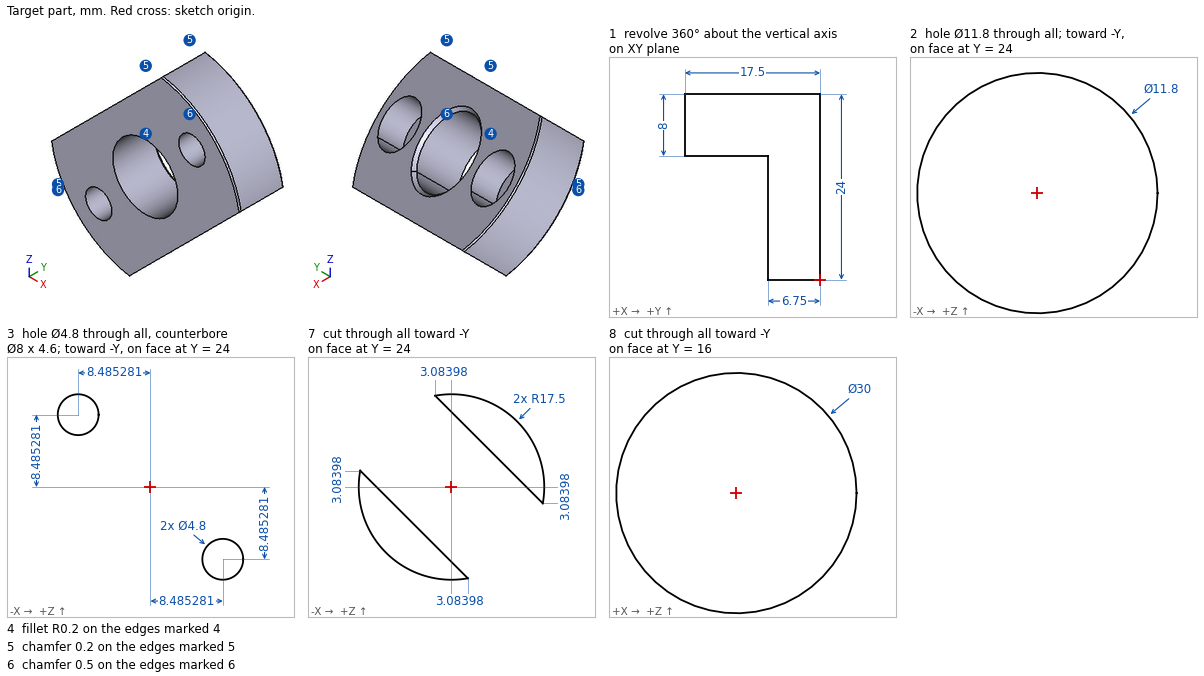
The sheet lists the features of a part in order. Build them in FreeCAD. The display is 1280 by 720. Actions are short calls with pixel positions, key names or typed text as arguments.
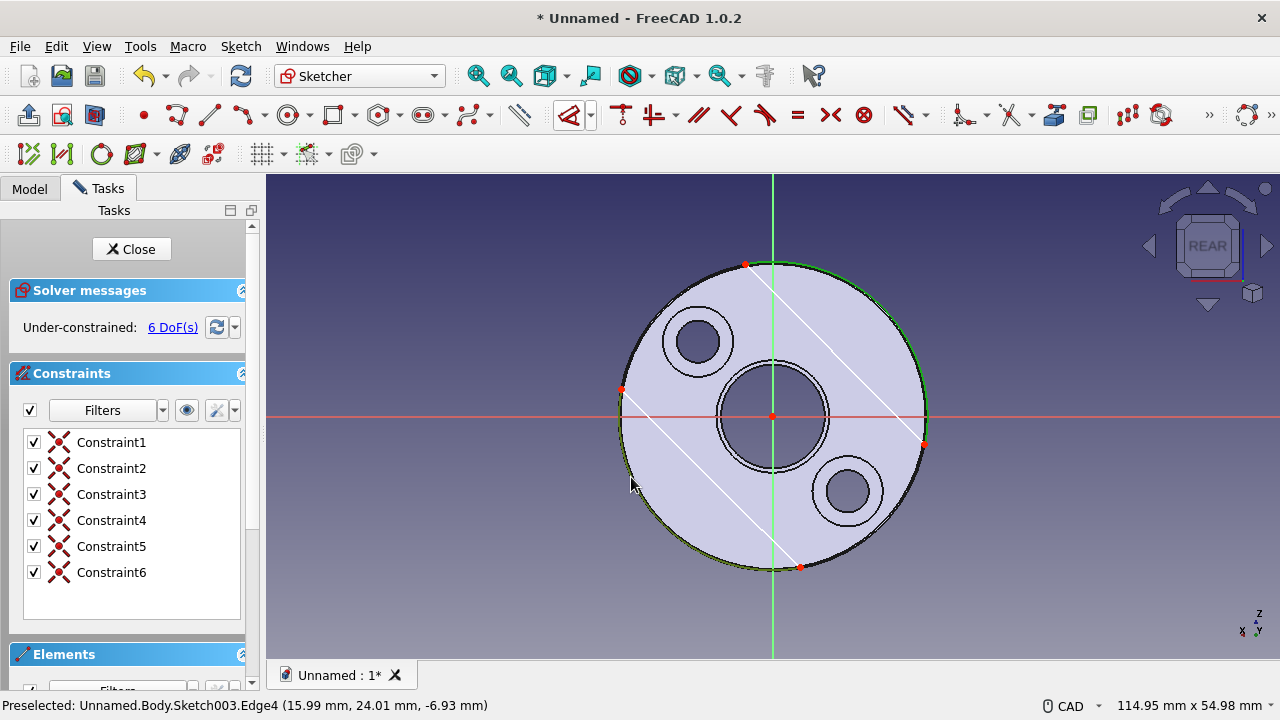
click(798, 116)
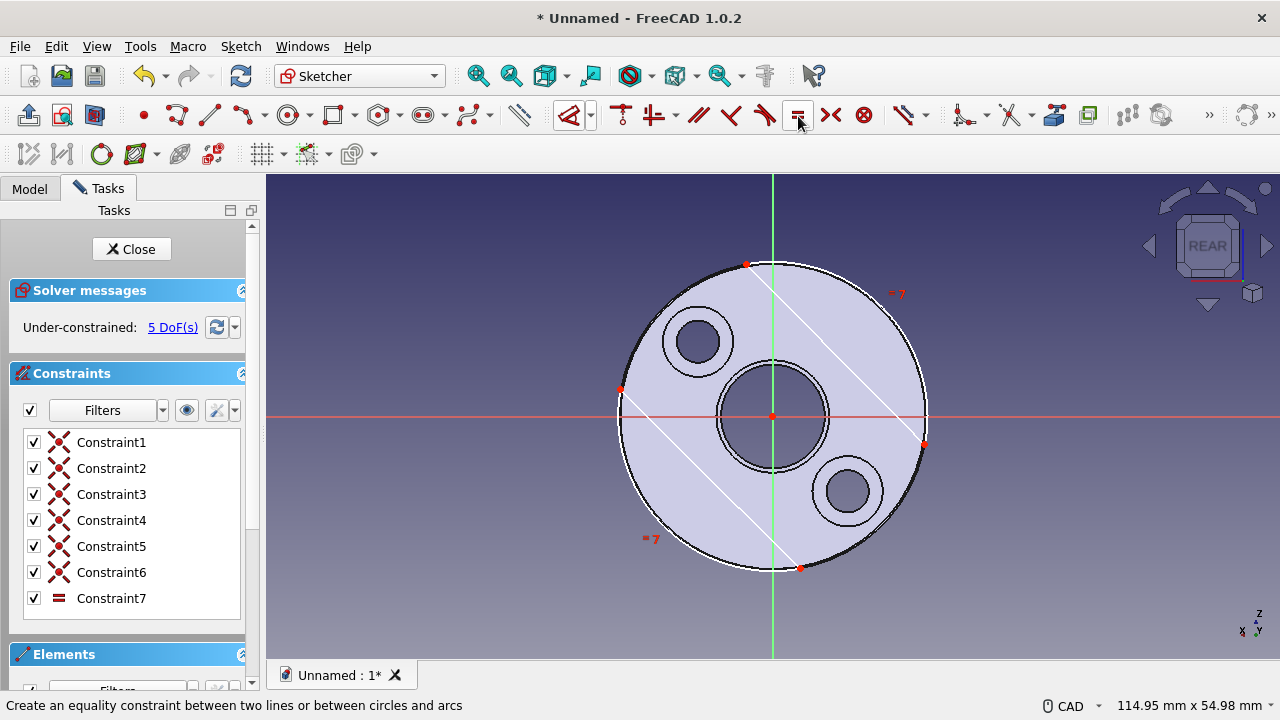
click(916, 357)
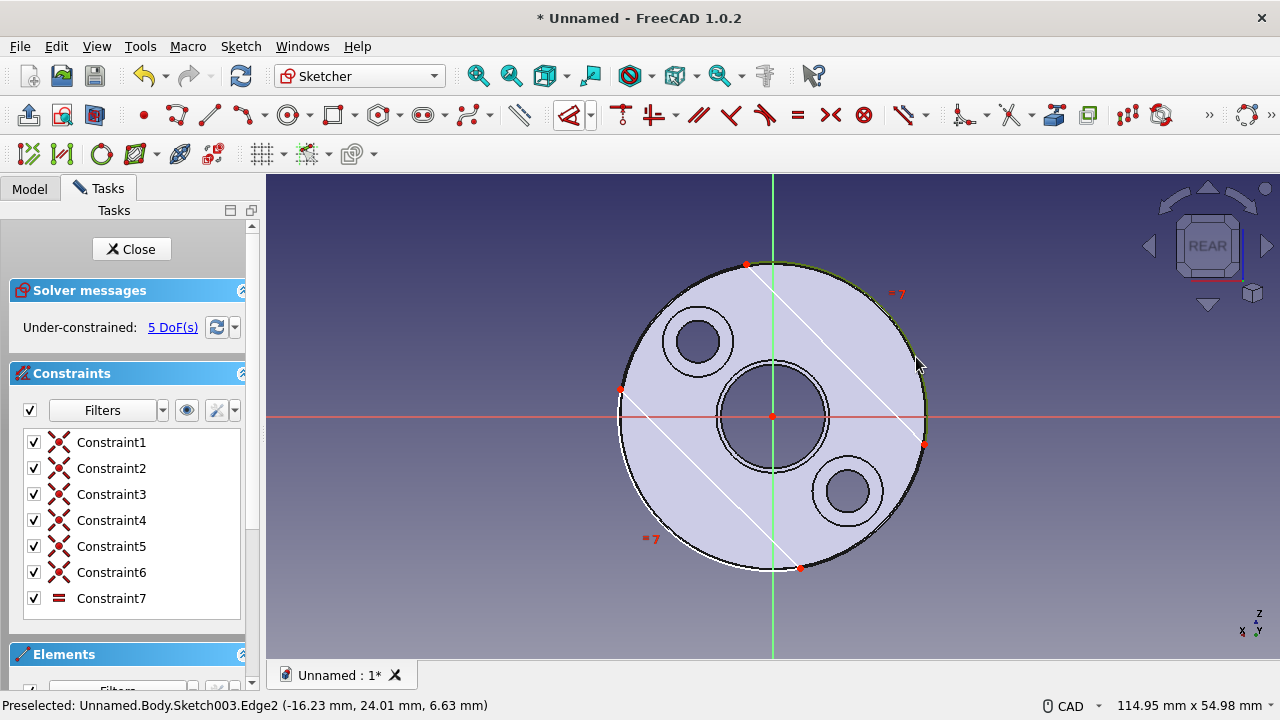
key(k)
key(r)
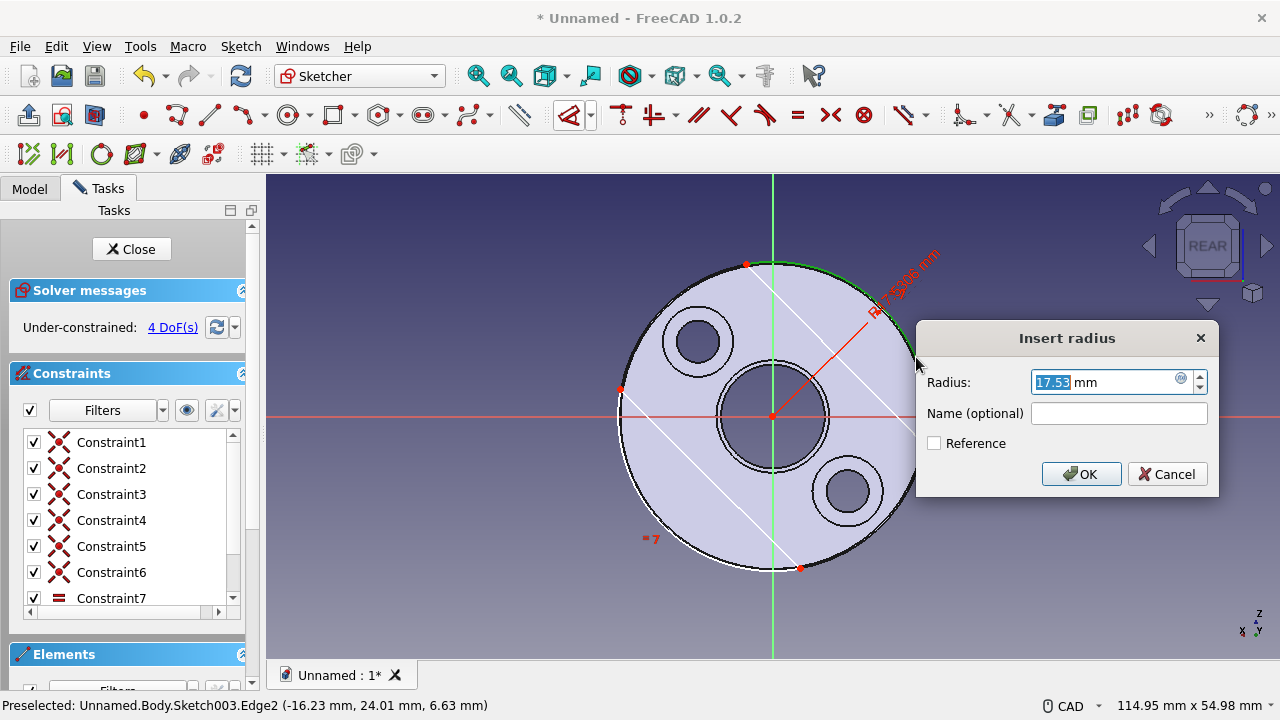
text(17.5)
key(Return)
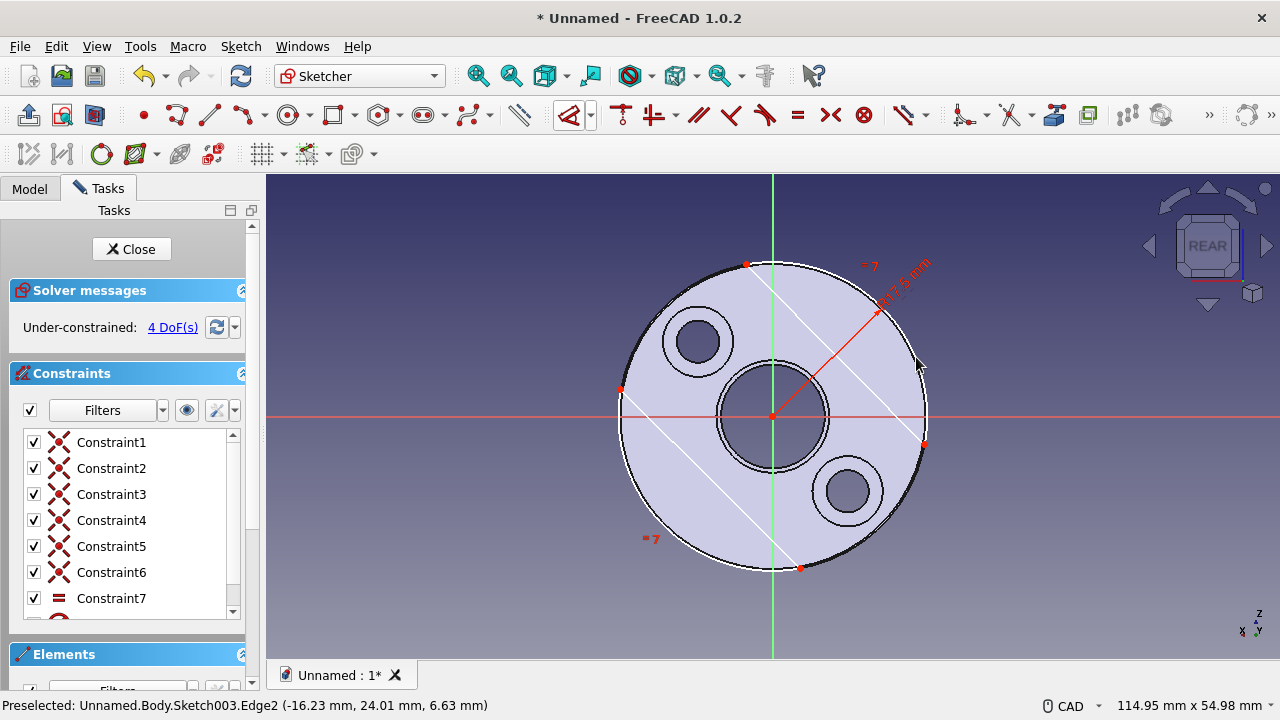
scroll(746, 264, up, 2)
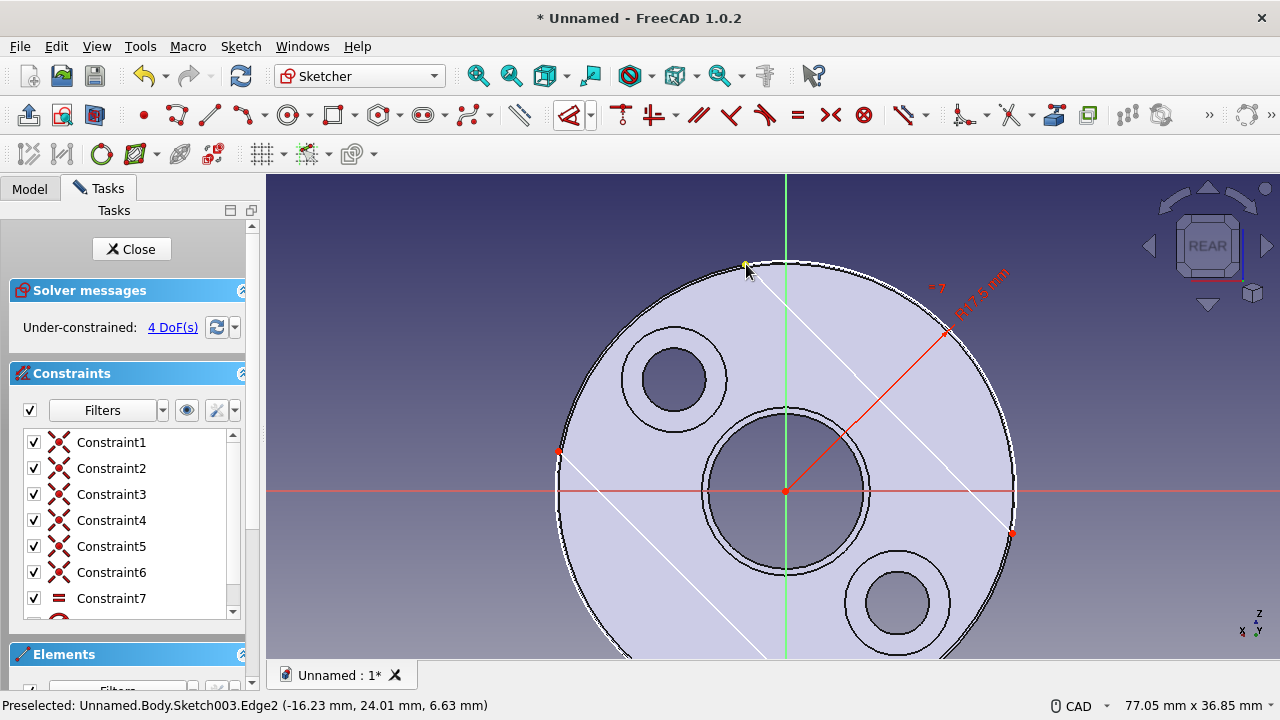
click(746, 265)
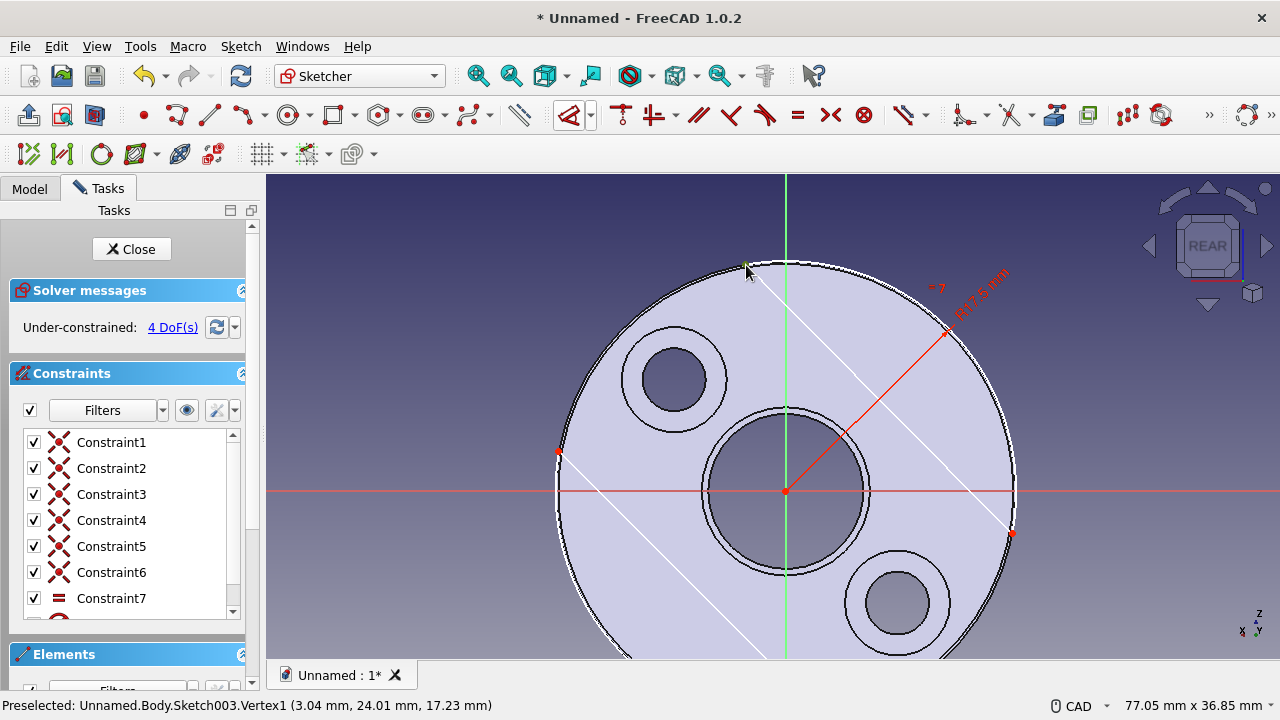
click(590, 116)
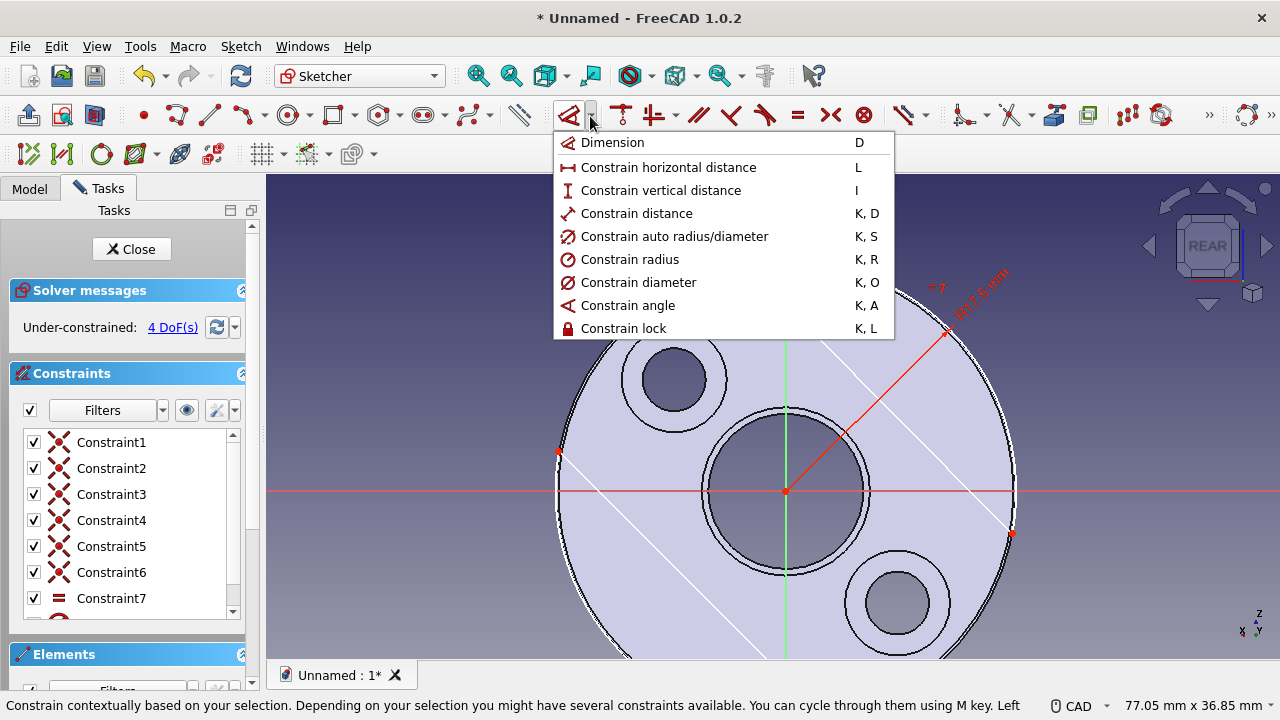
click(724, 168)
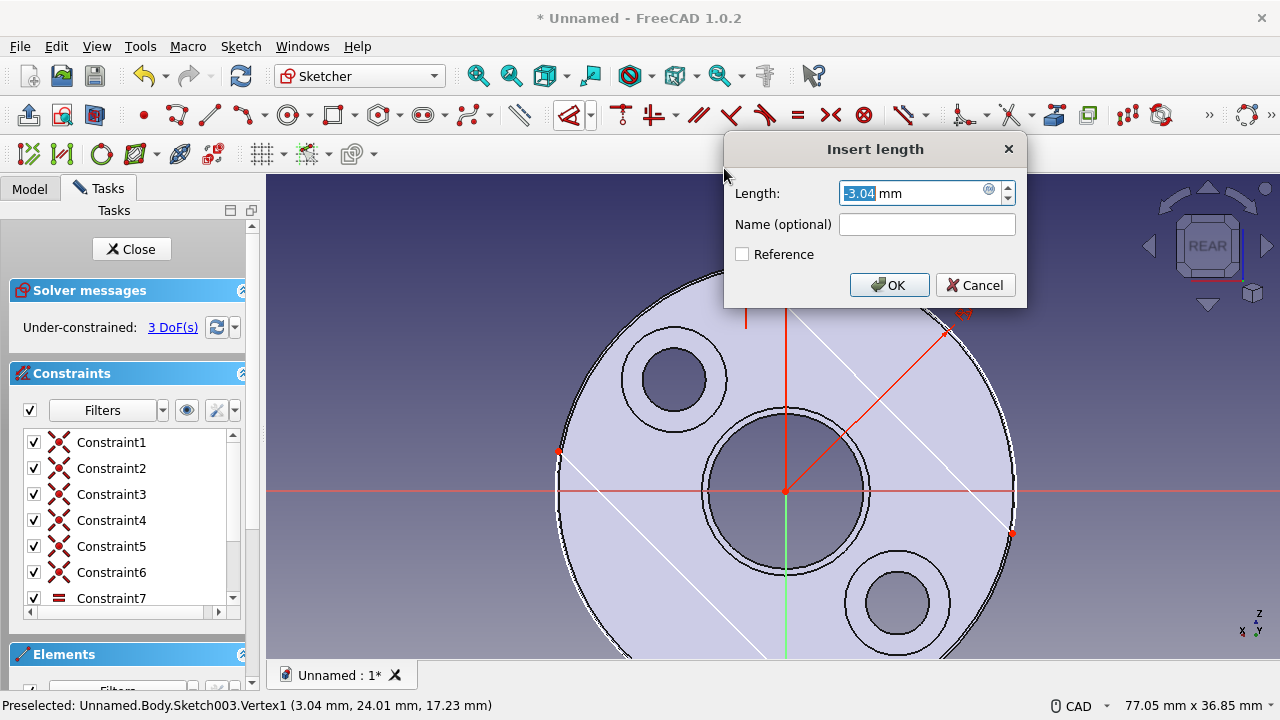
text(-3.08398)
key(Return)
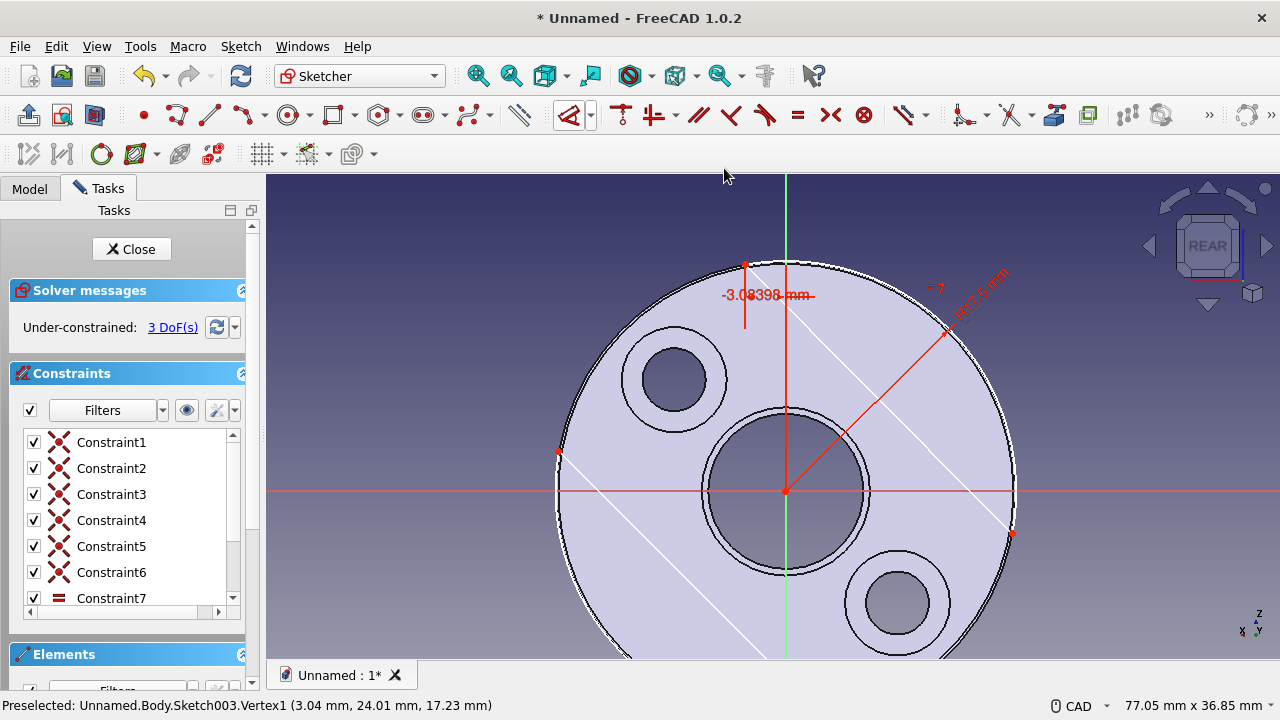
click(1012, 534)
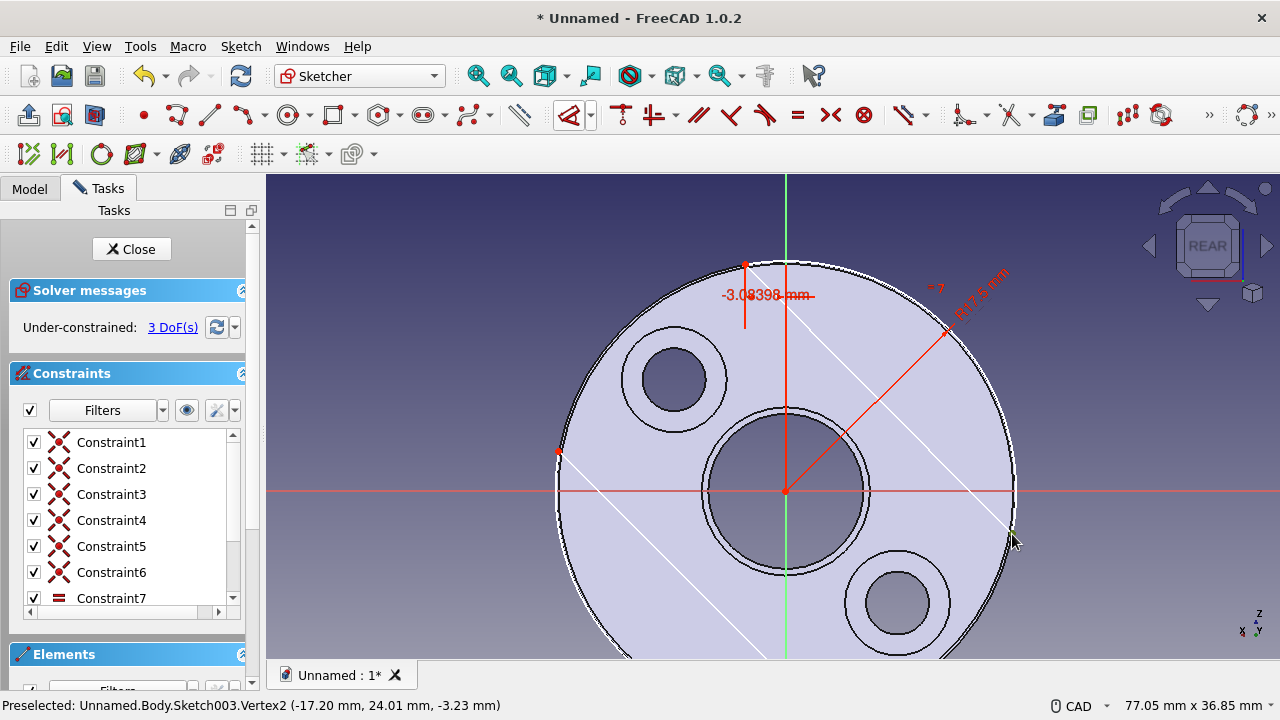
key(i)